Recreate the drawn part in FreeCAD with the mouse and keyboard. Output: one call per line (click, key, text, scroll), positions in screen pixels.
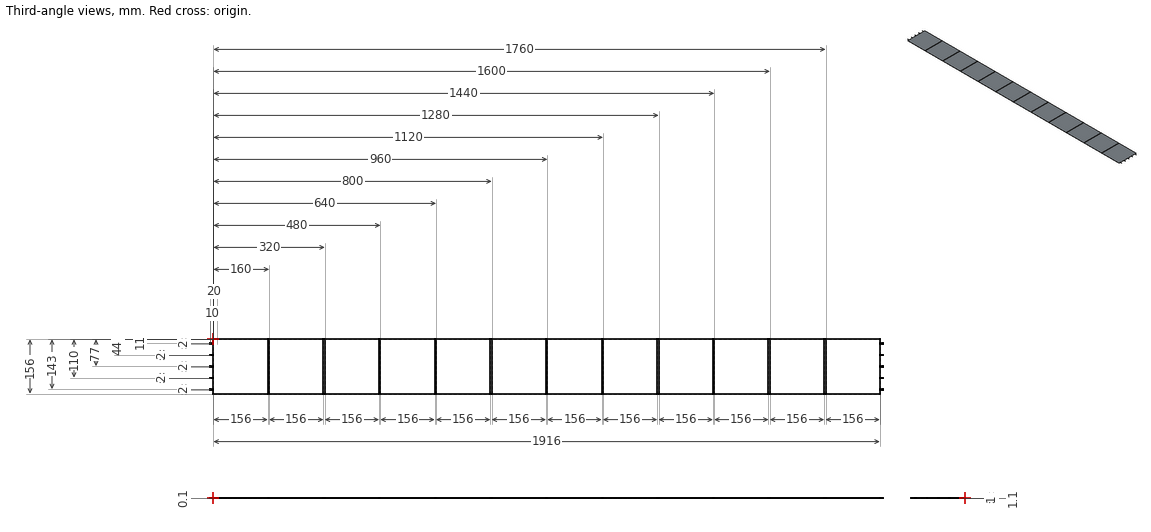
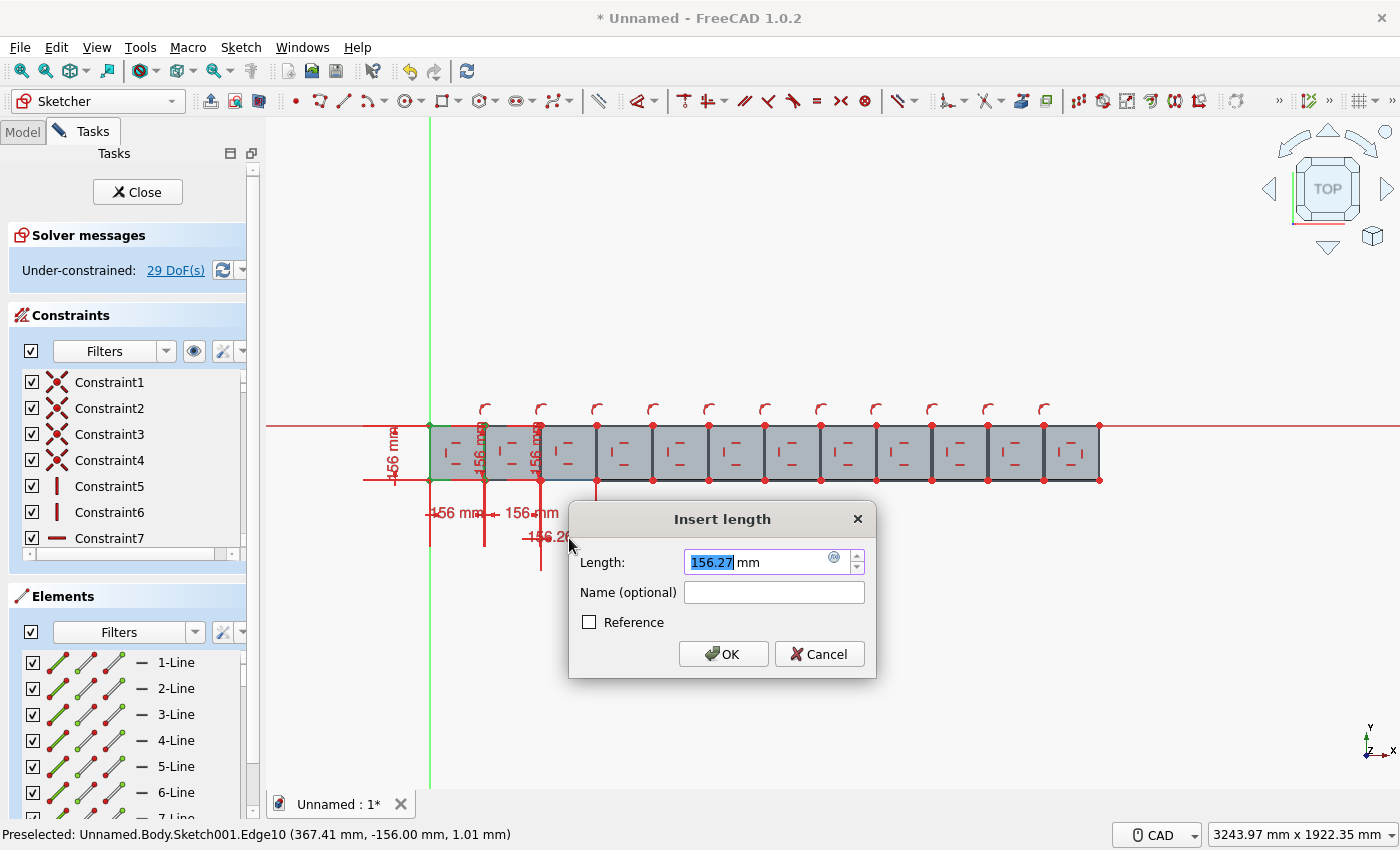
text(156)
key(Return)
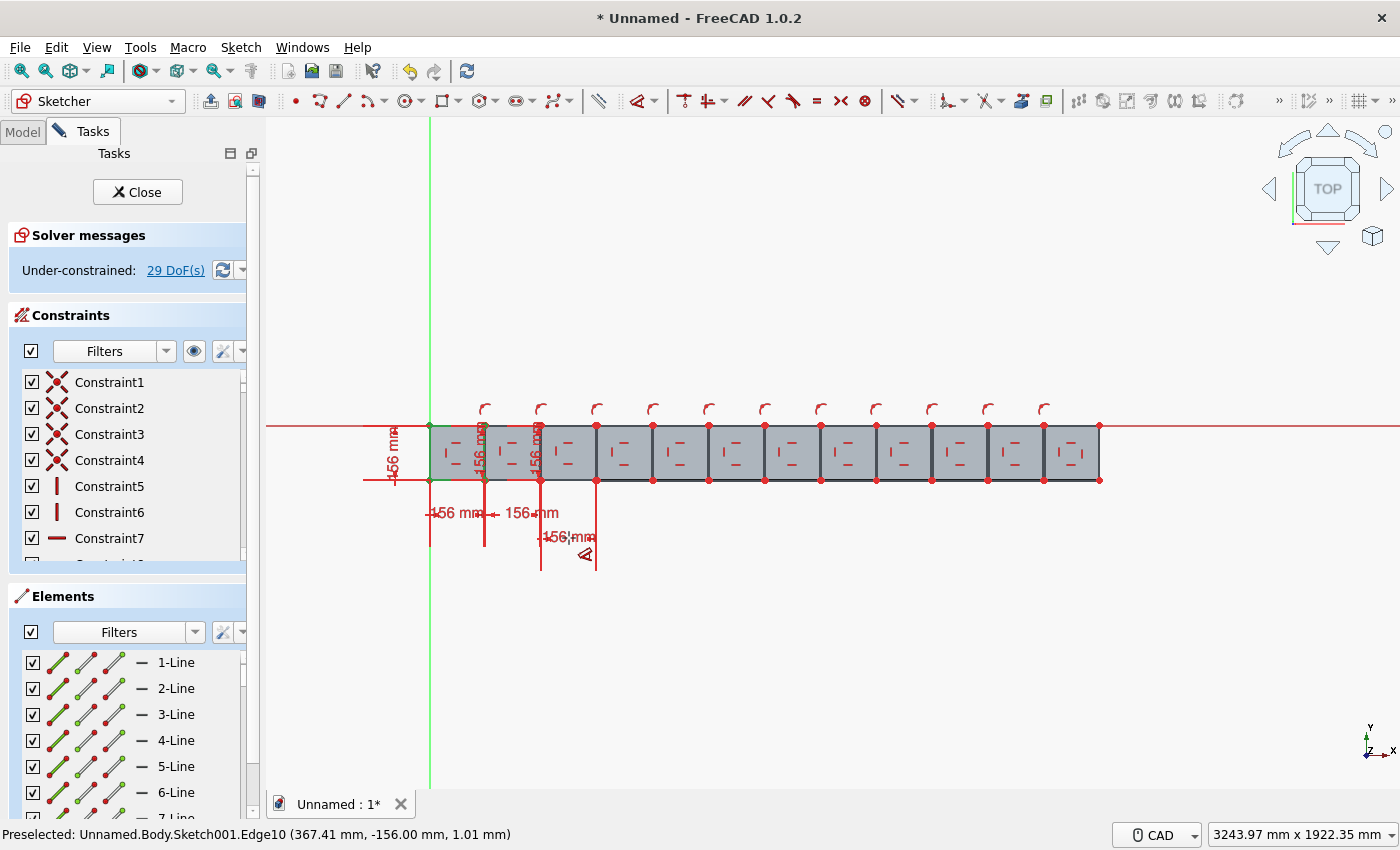
scroll(597, 442, up, 12)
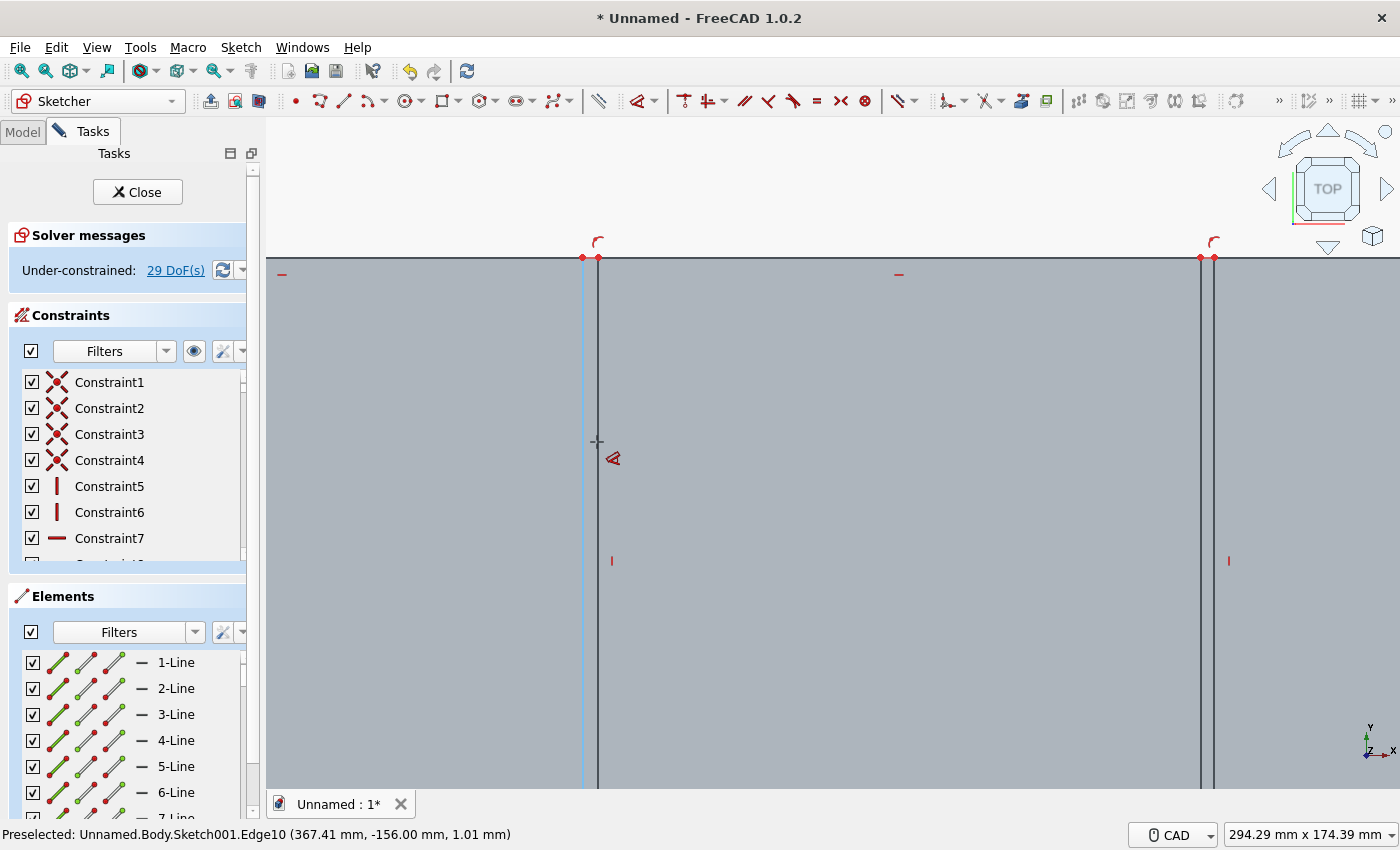
click(598, 441)
click(564, 509)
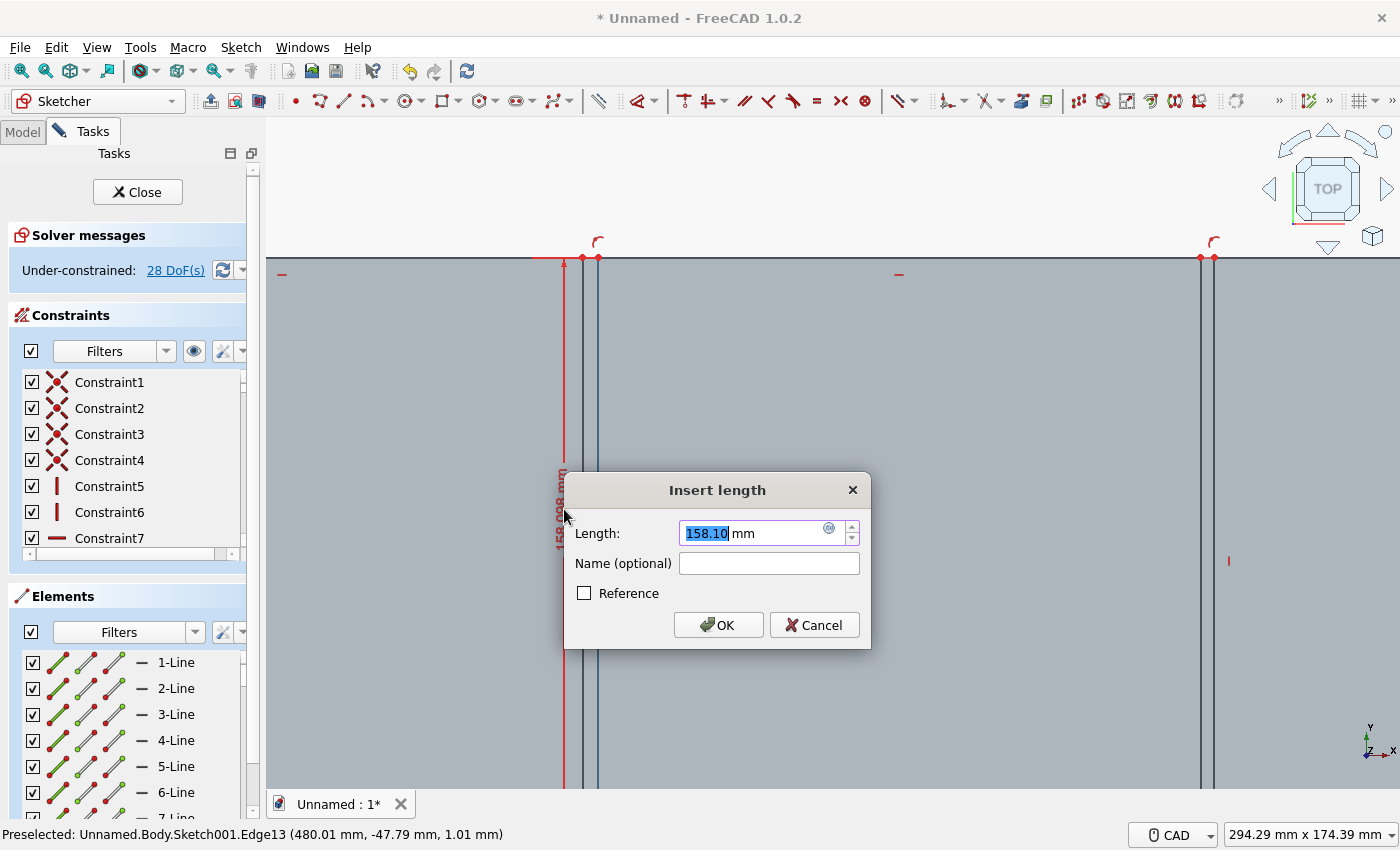
text(156)
key(Return)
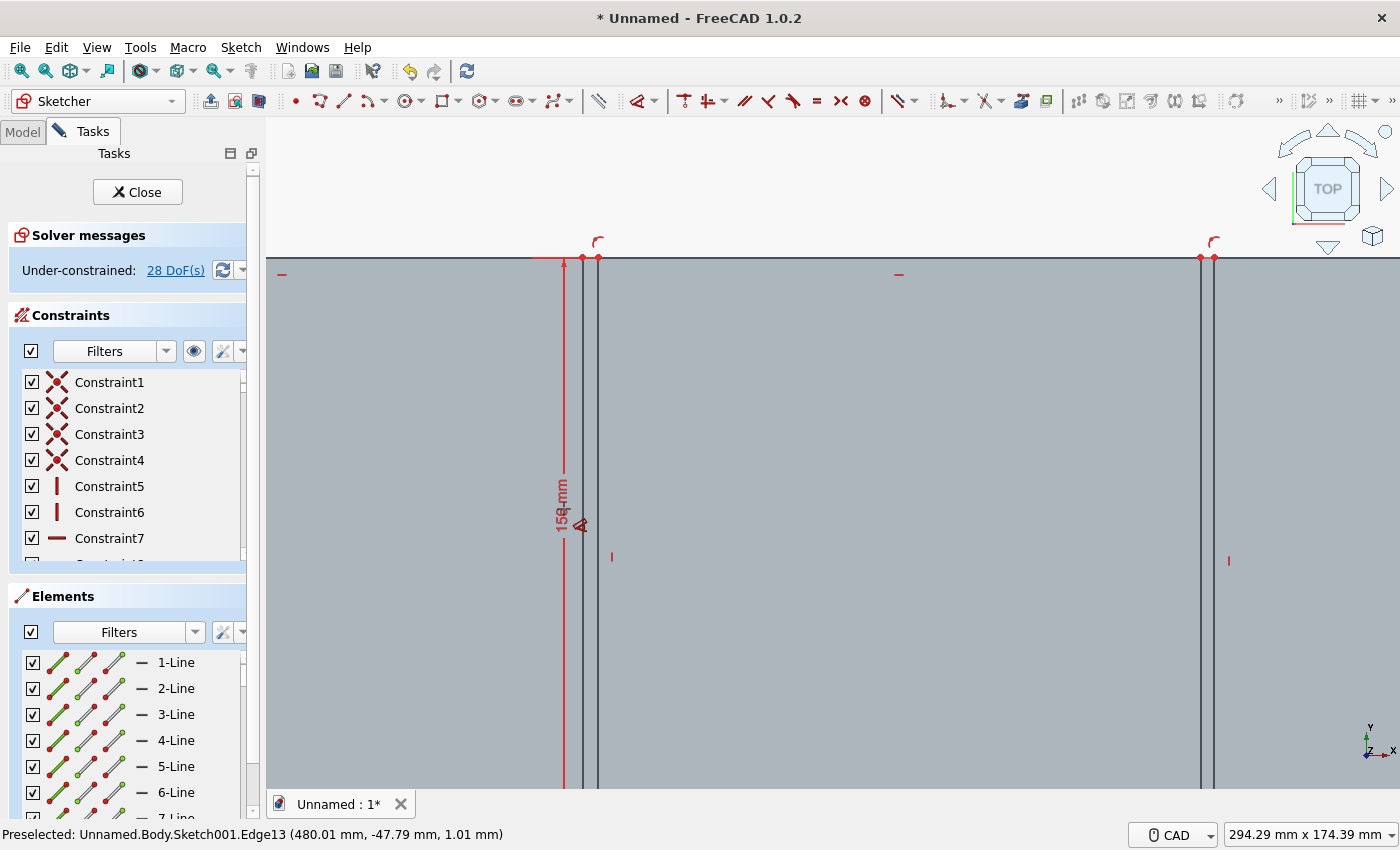
scroll(597, 442, down, 12)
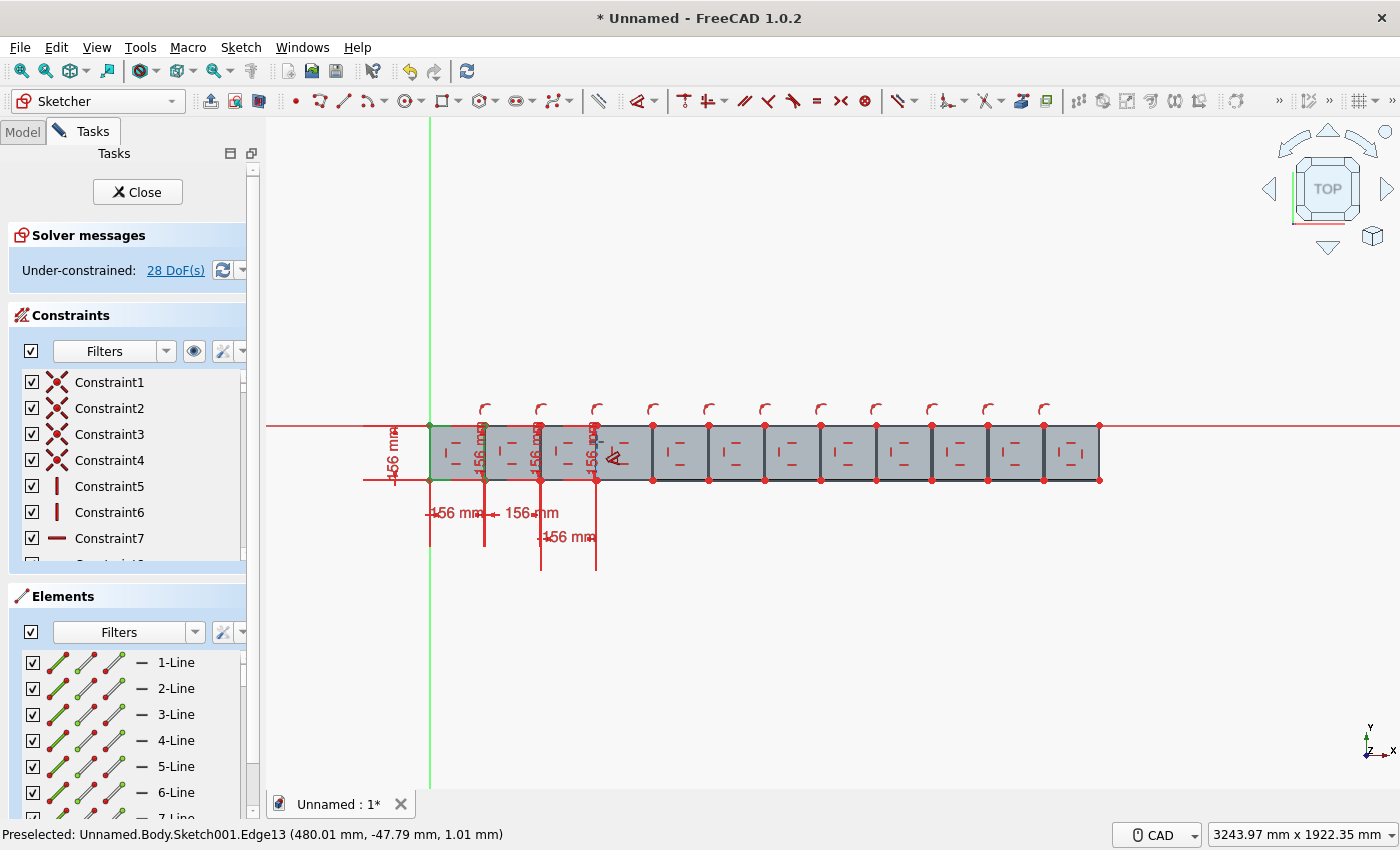
click(614, 480)
click(625, 514)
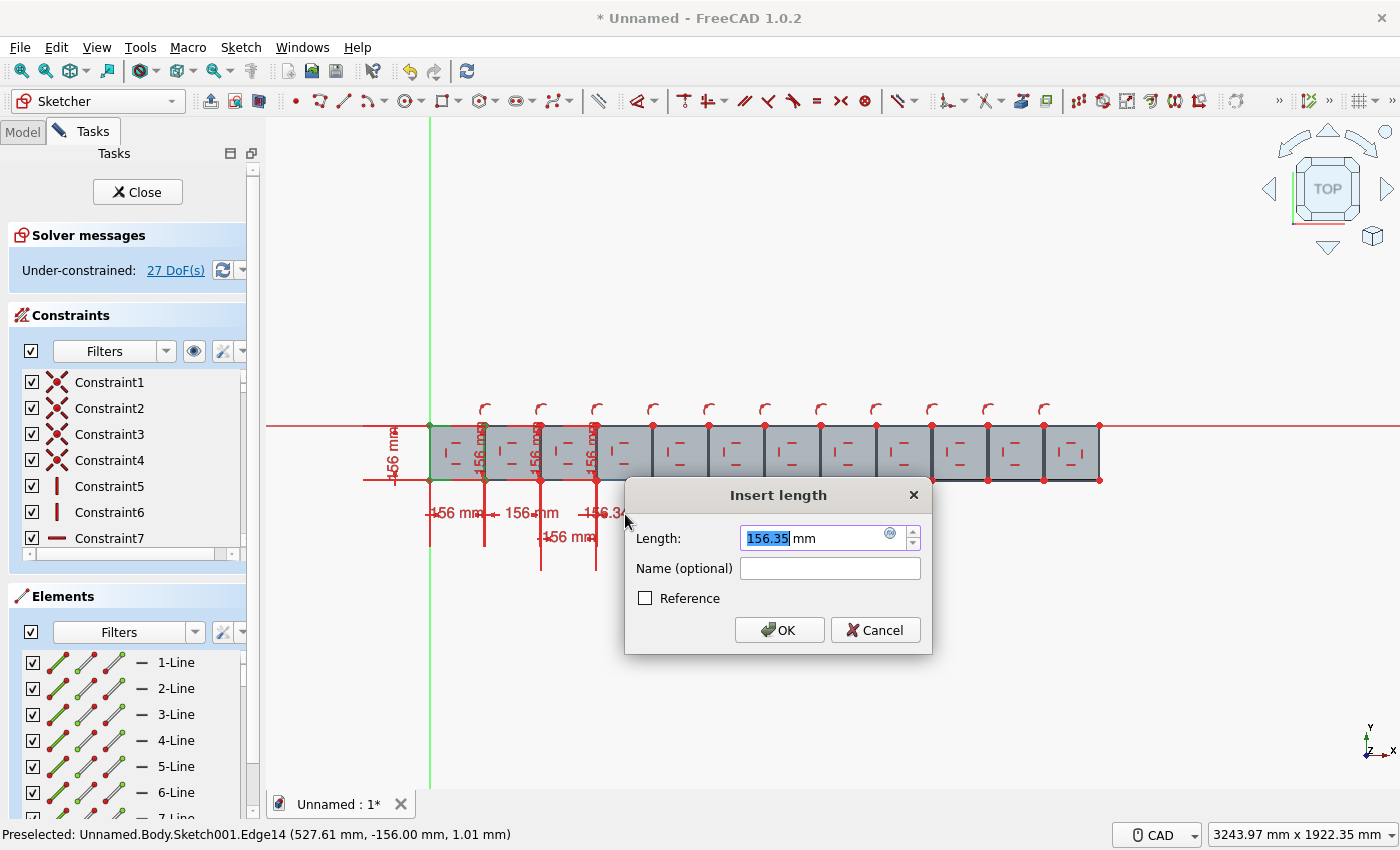
text(156)
key(Return)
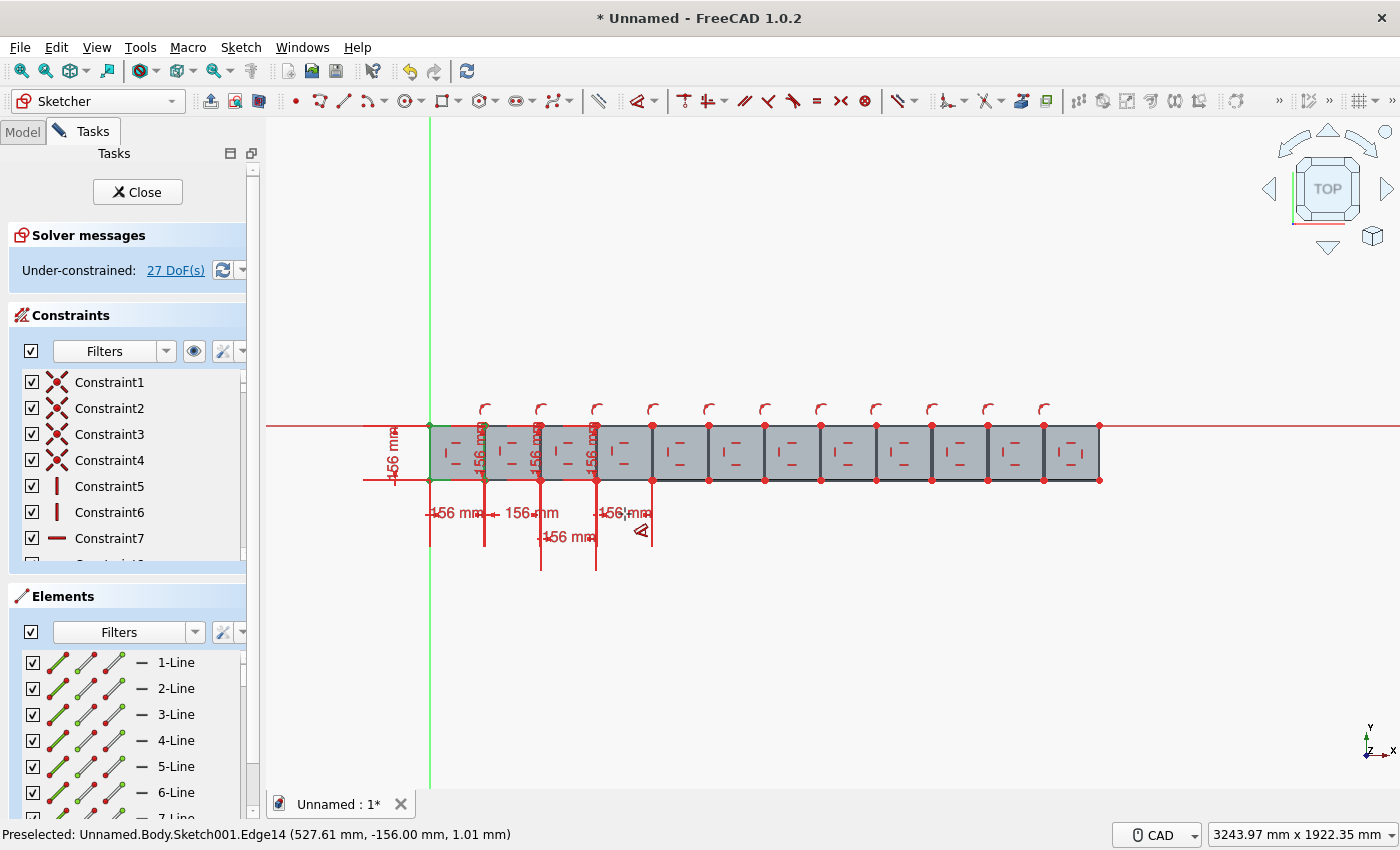
scroll(653, 442, up, 12)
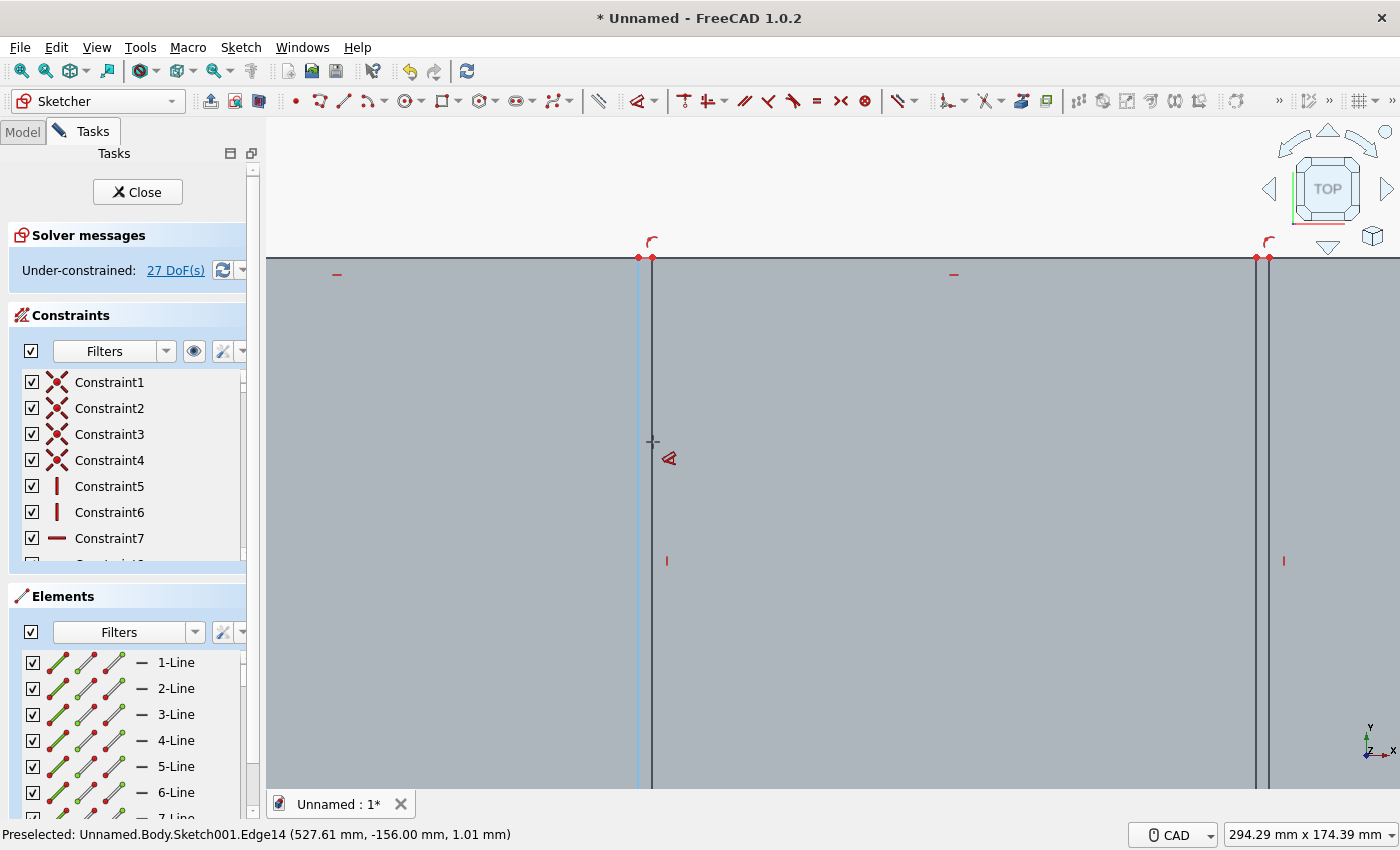
click(652, 441)
click(618, 509)